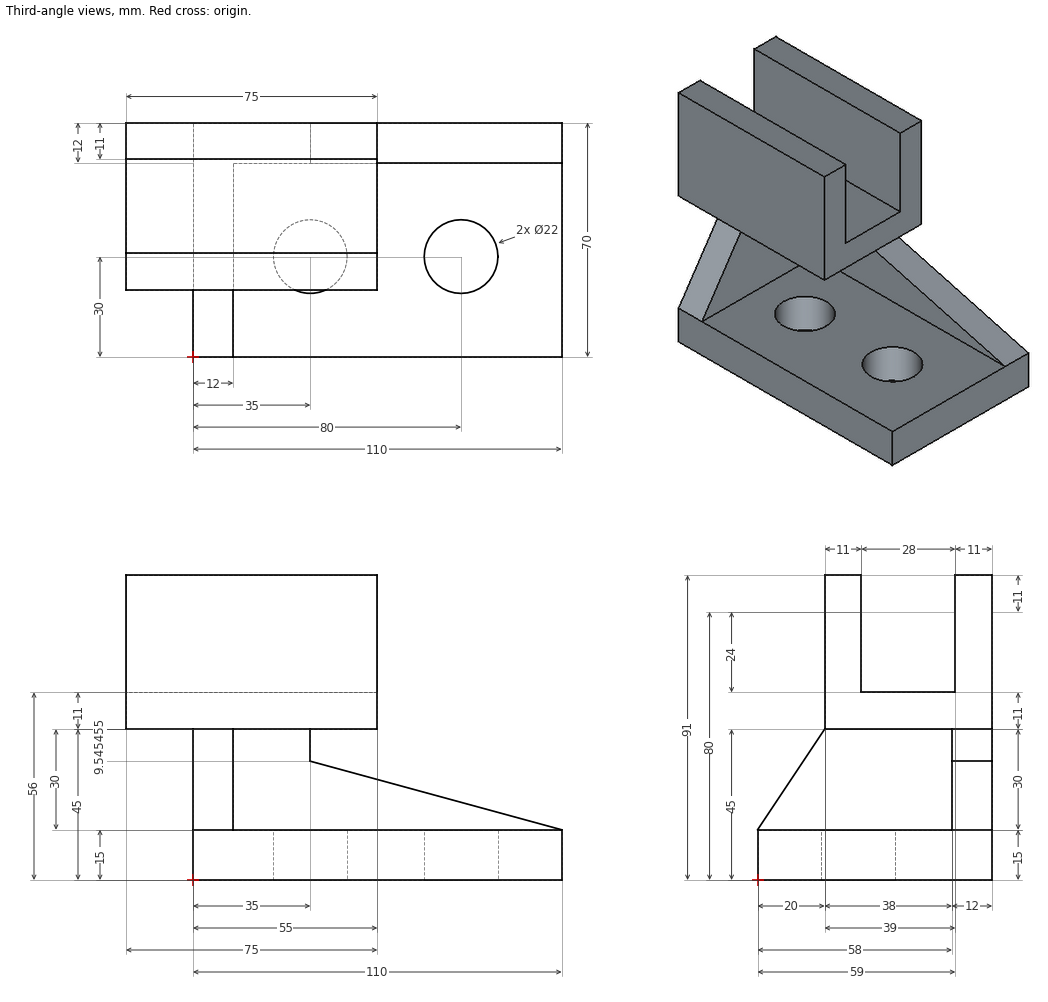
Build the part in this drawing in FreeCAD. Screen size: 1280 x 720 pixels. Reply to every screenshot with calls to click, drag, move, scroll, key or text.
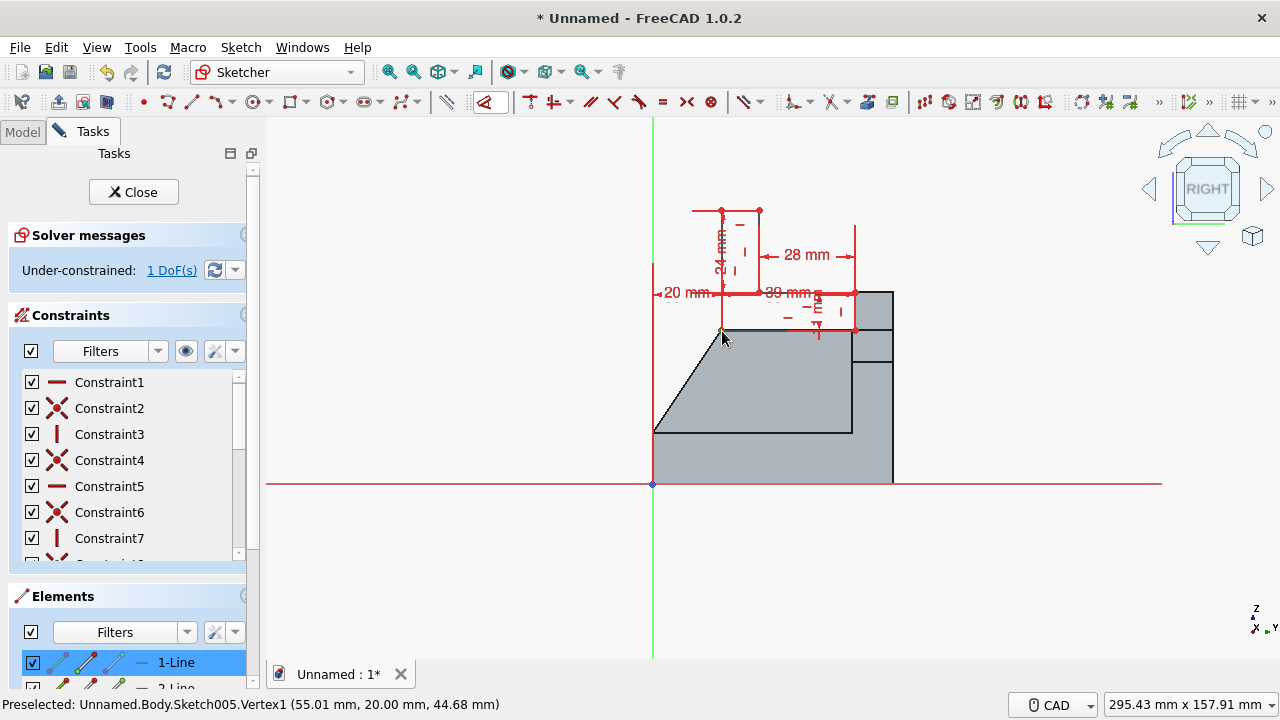
key(i)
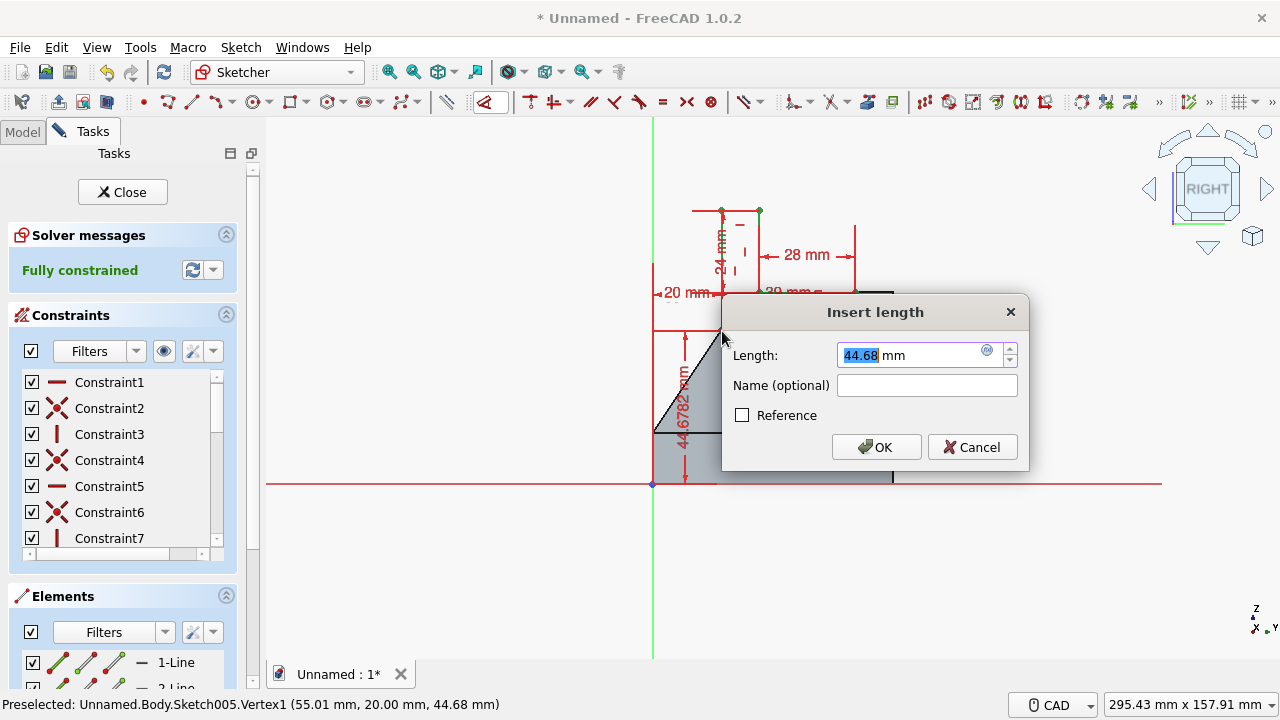
text(45)
key(Return)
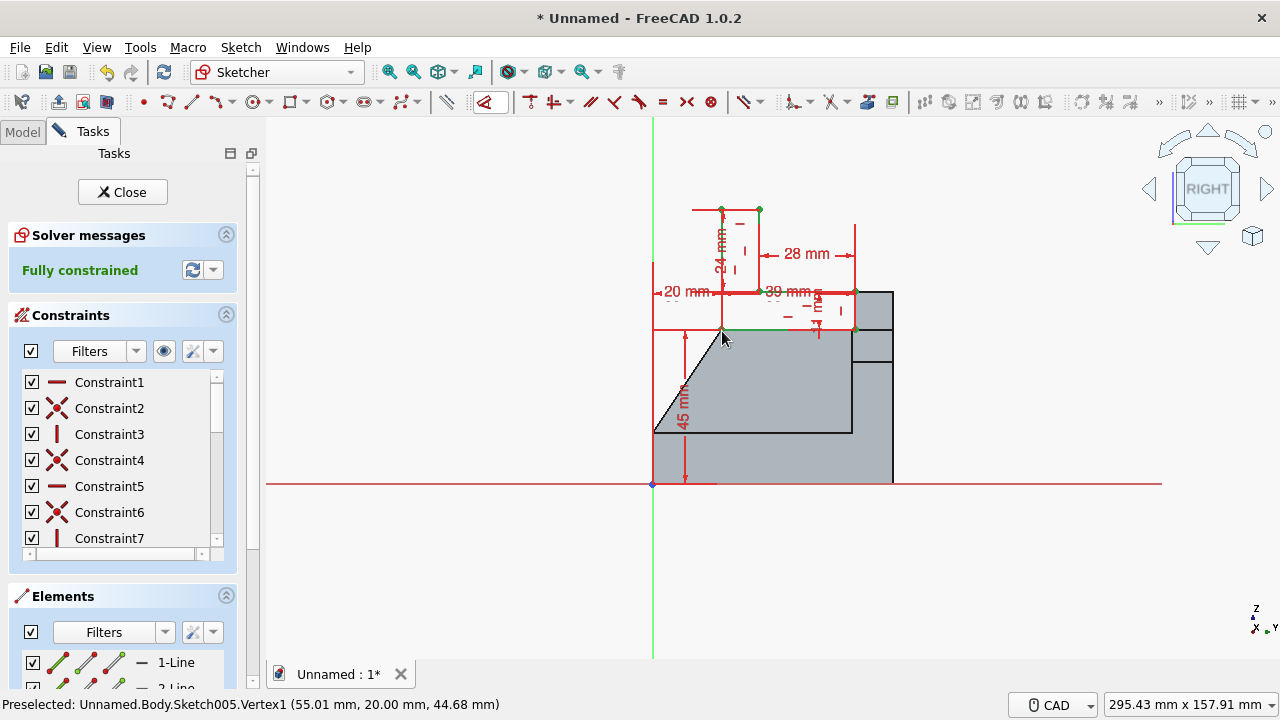
click(123, 192)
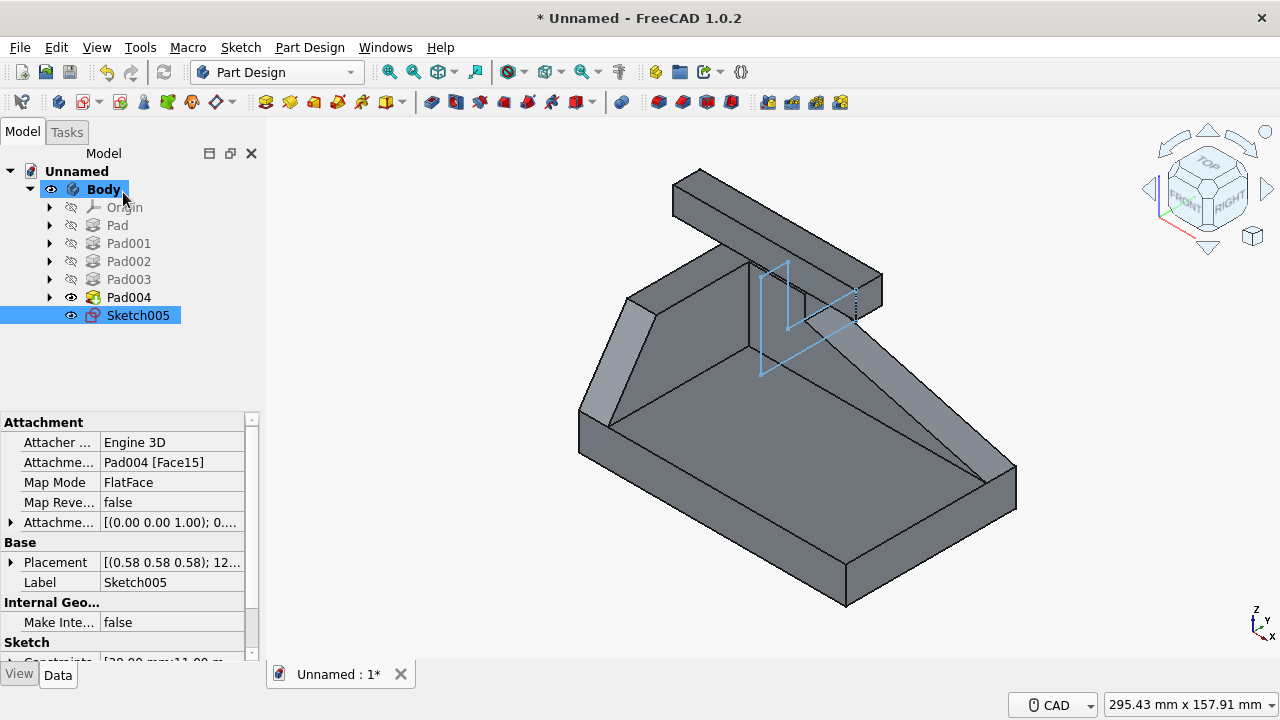
click(266, 102)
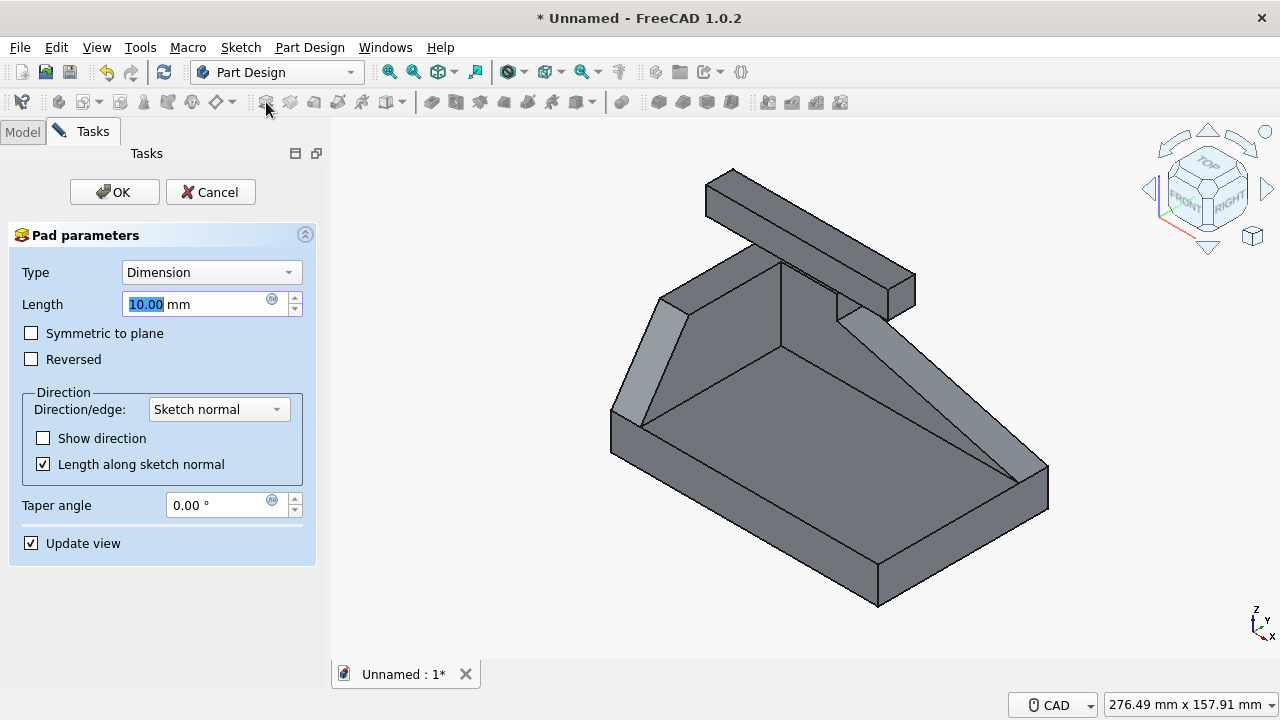
text(75)
key(Tab)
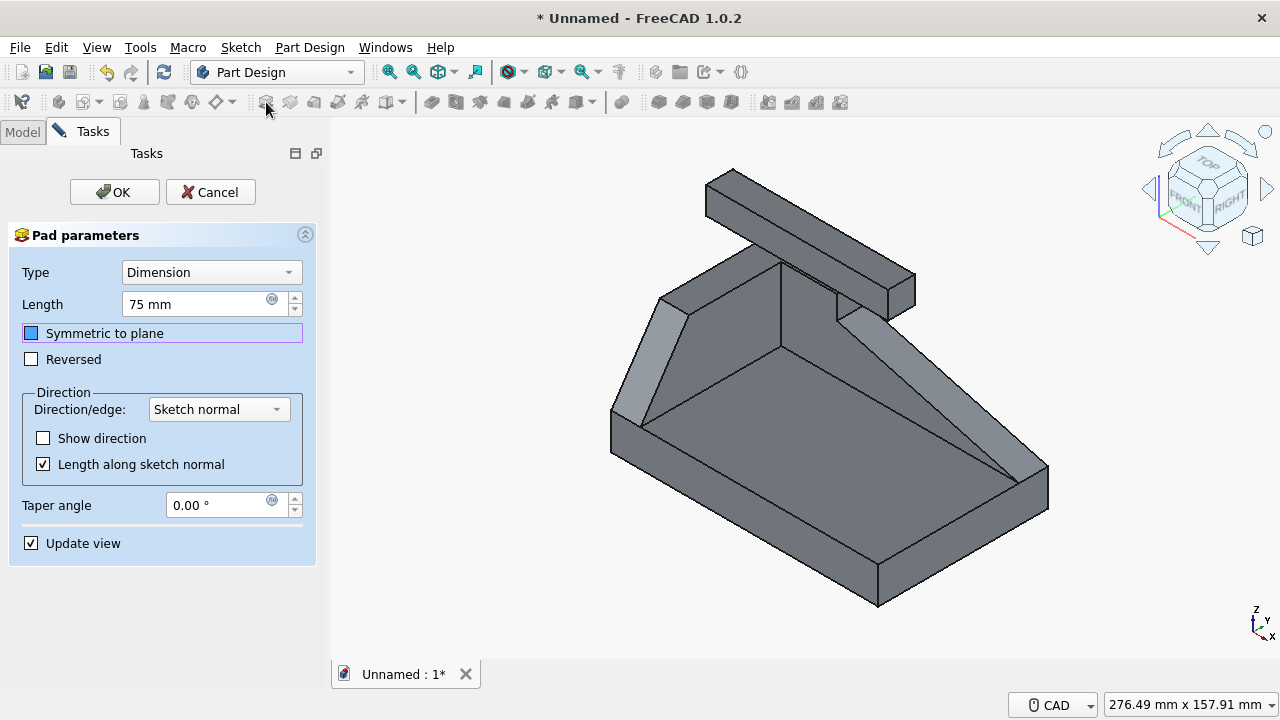
click(30, 359)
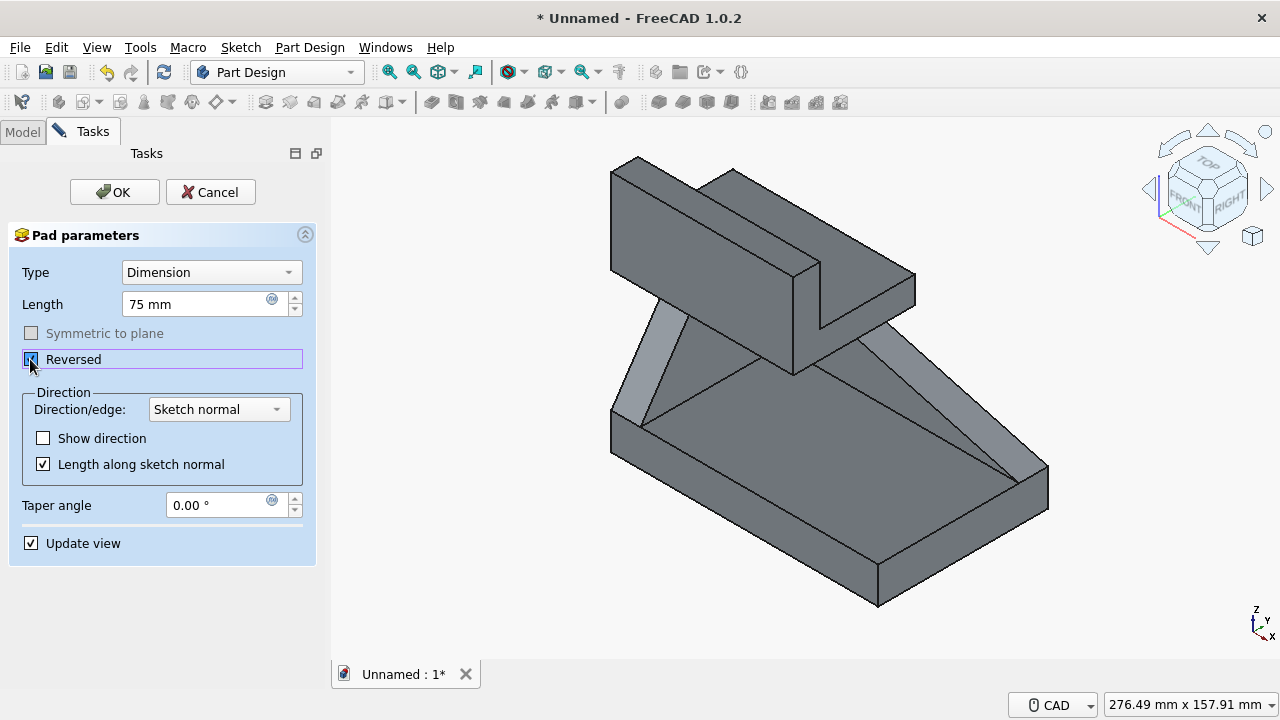
click(115, 192)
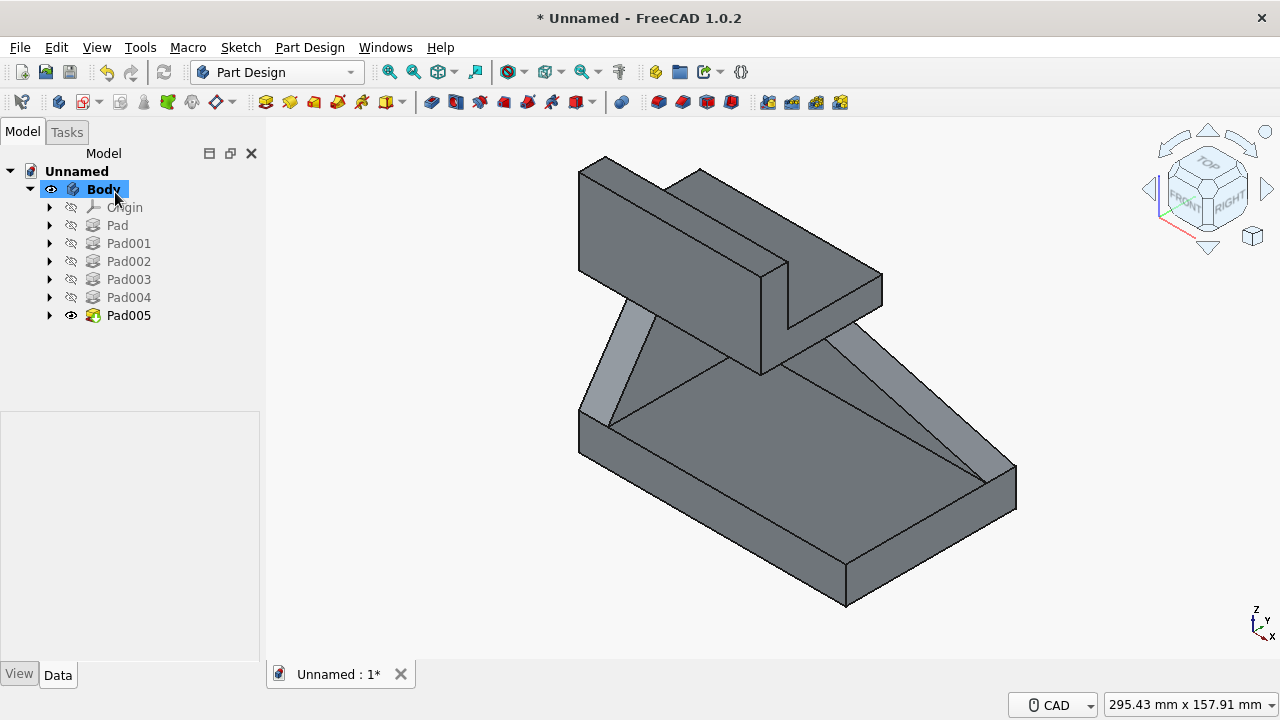
click(390, 72)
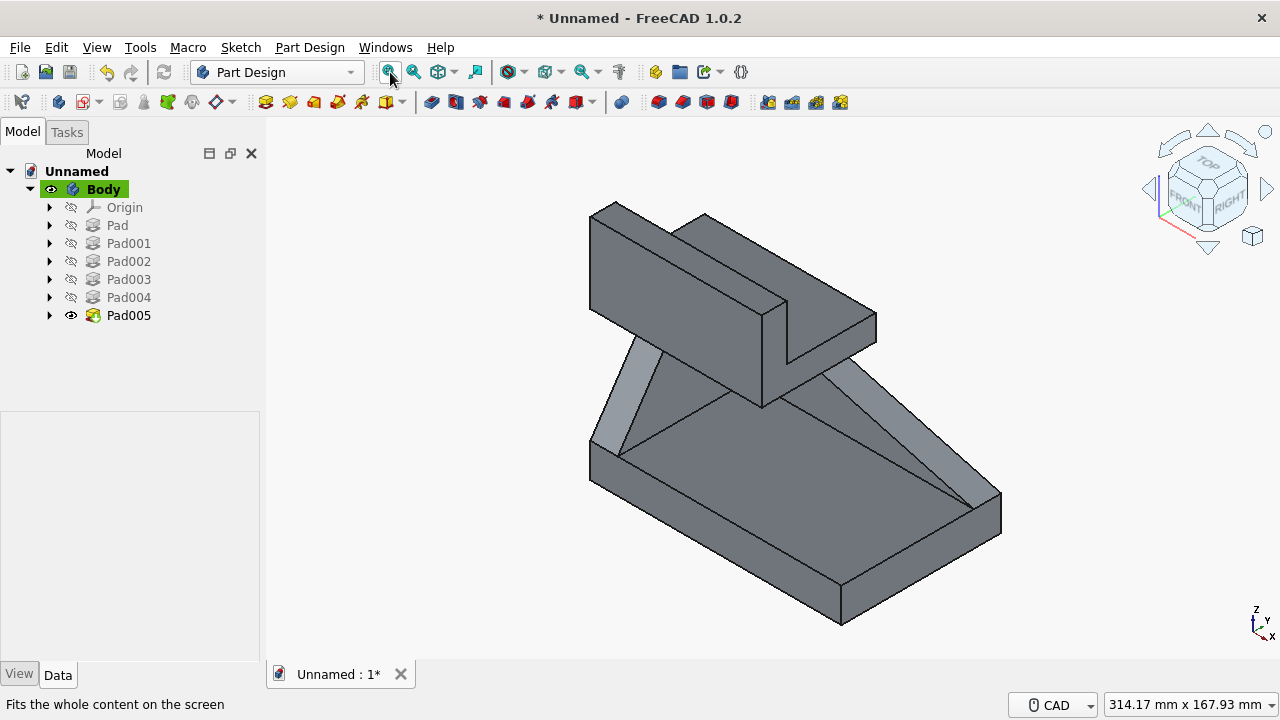
click(770, 330)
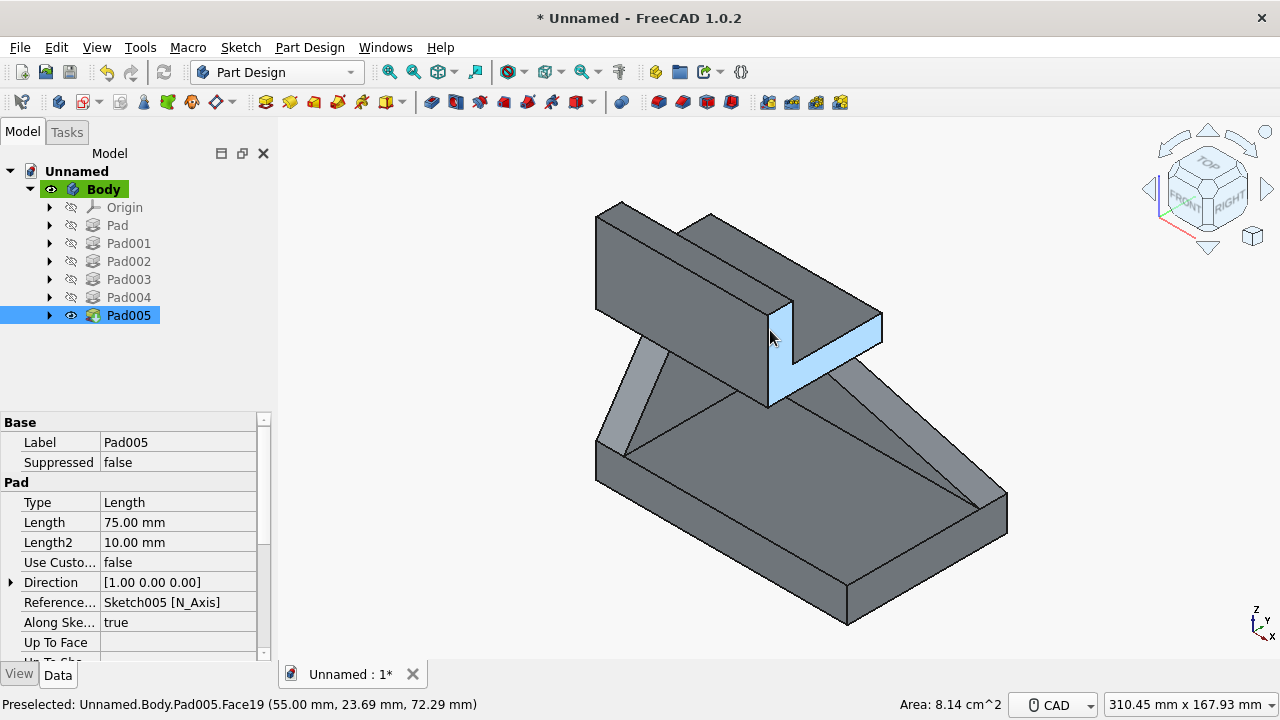
click(84, 102)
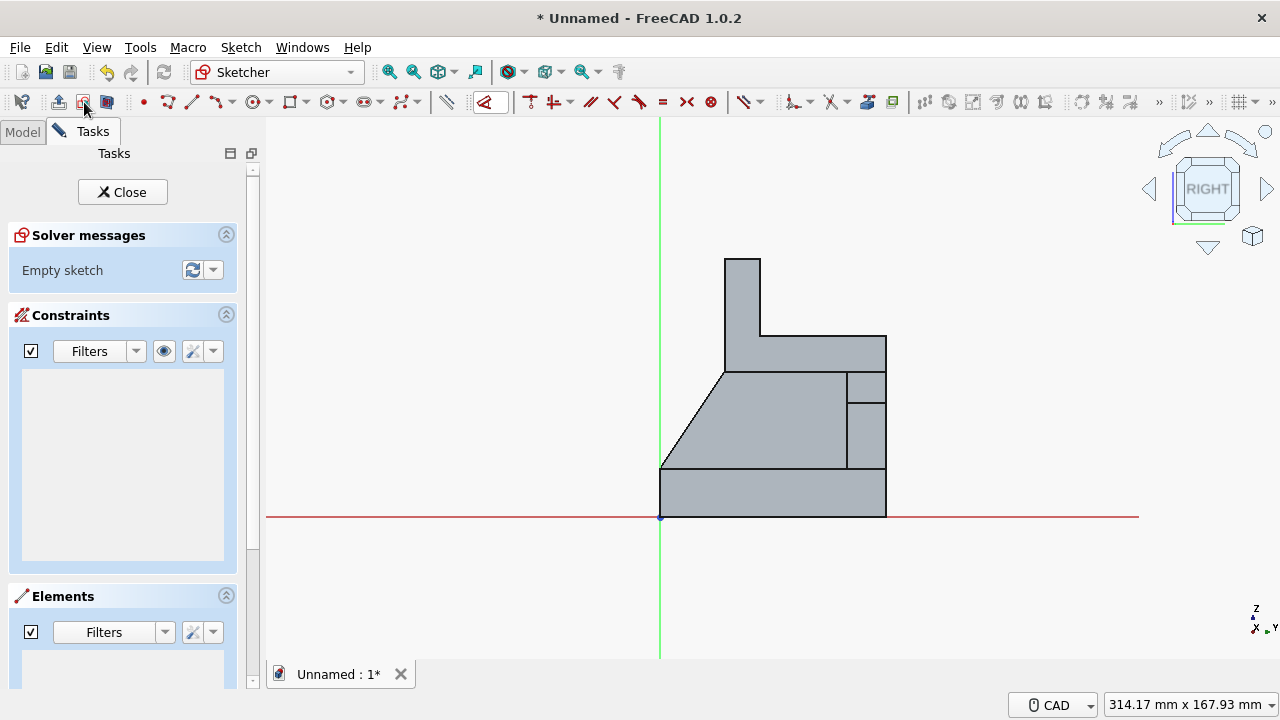
scroll(922, 268, up, 7)